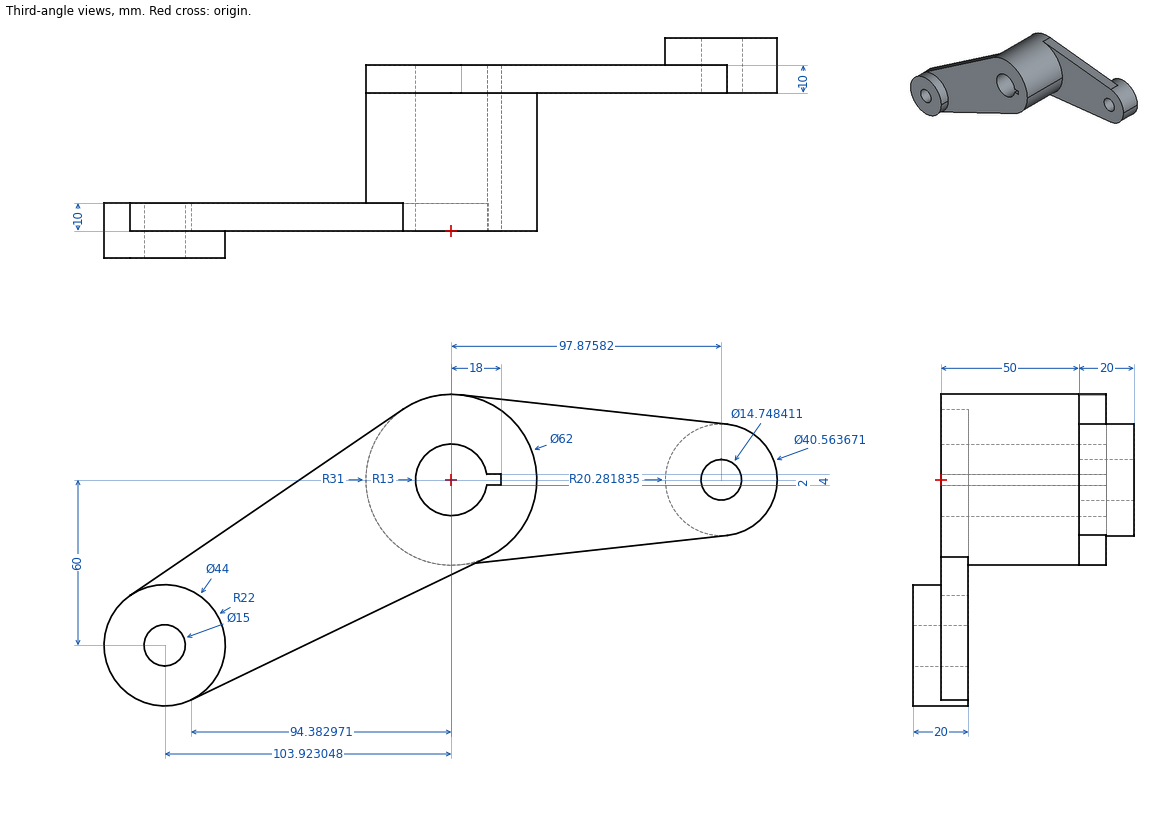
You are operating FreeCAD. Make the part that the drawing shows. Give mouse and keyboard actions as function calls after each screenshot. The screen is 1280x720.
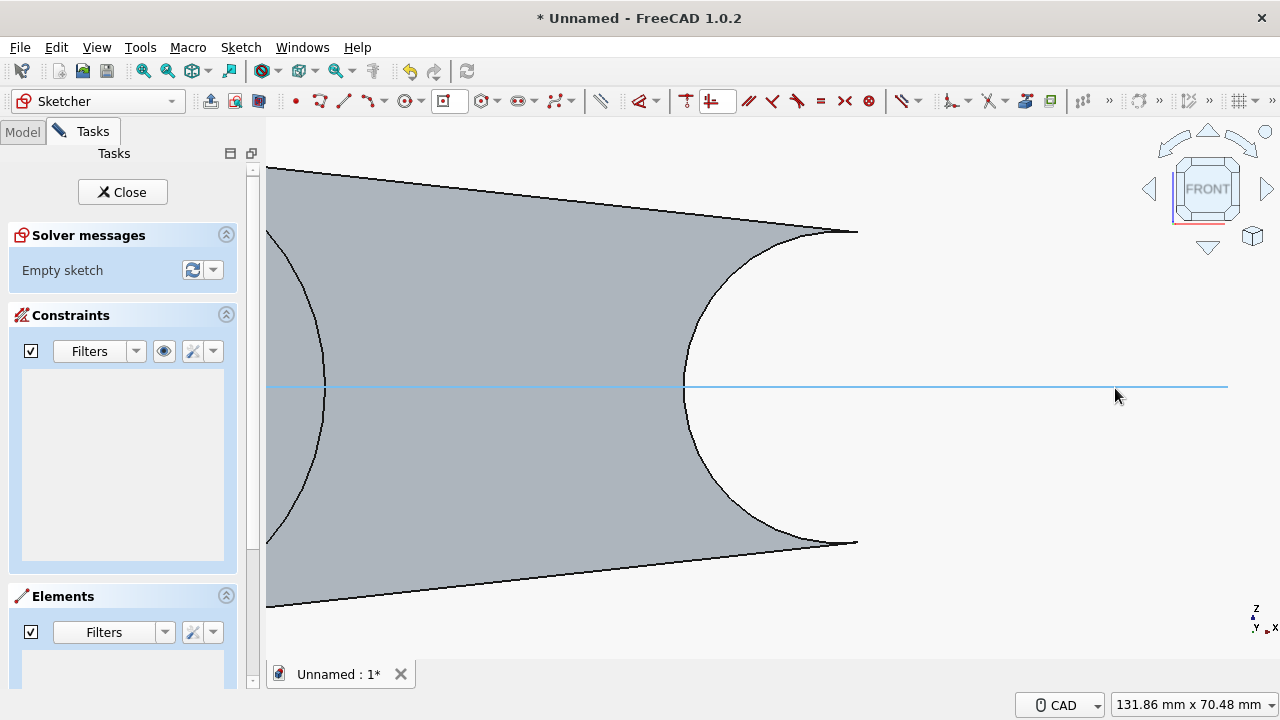
click(406, 102)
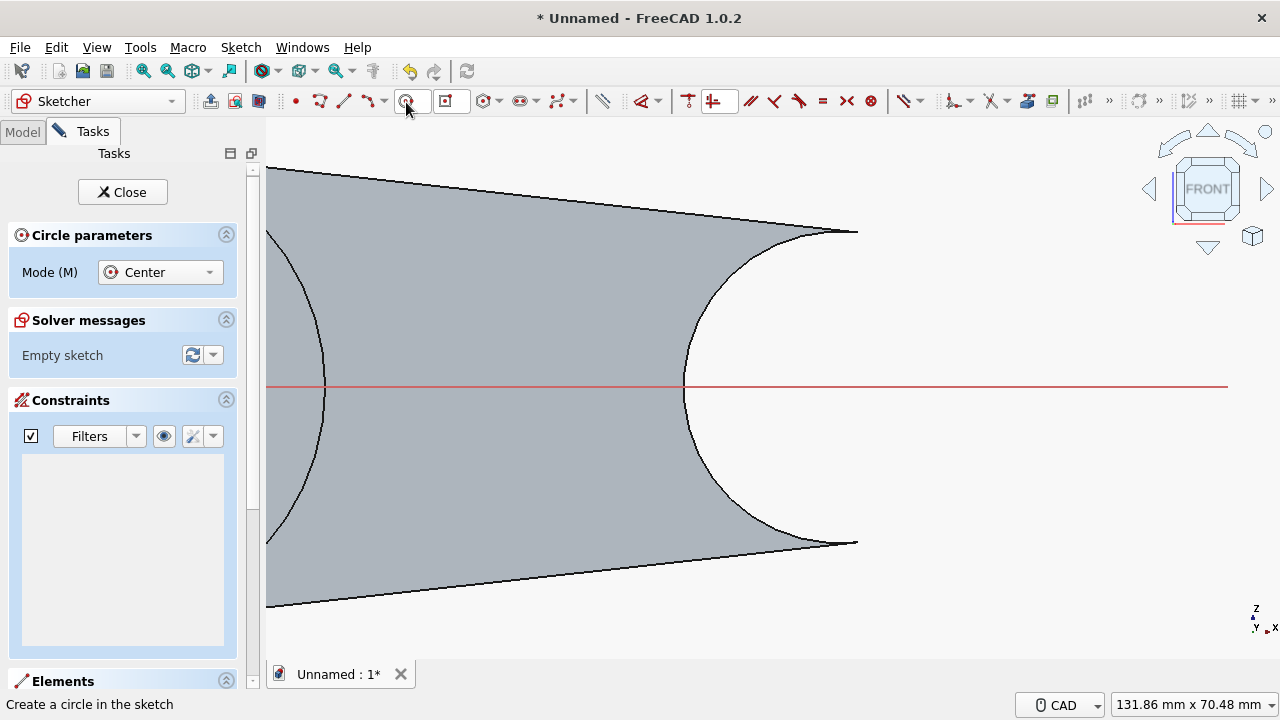
click(840, 387)
move(950, 277)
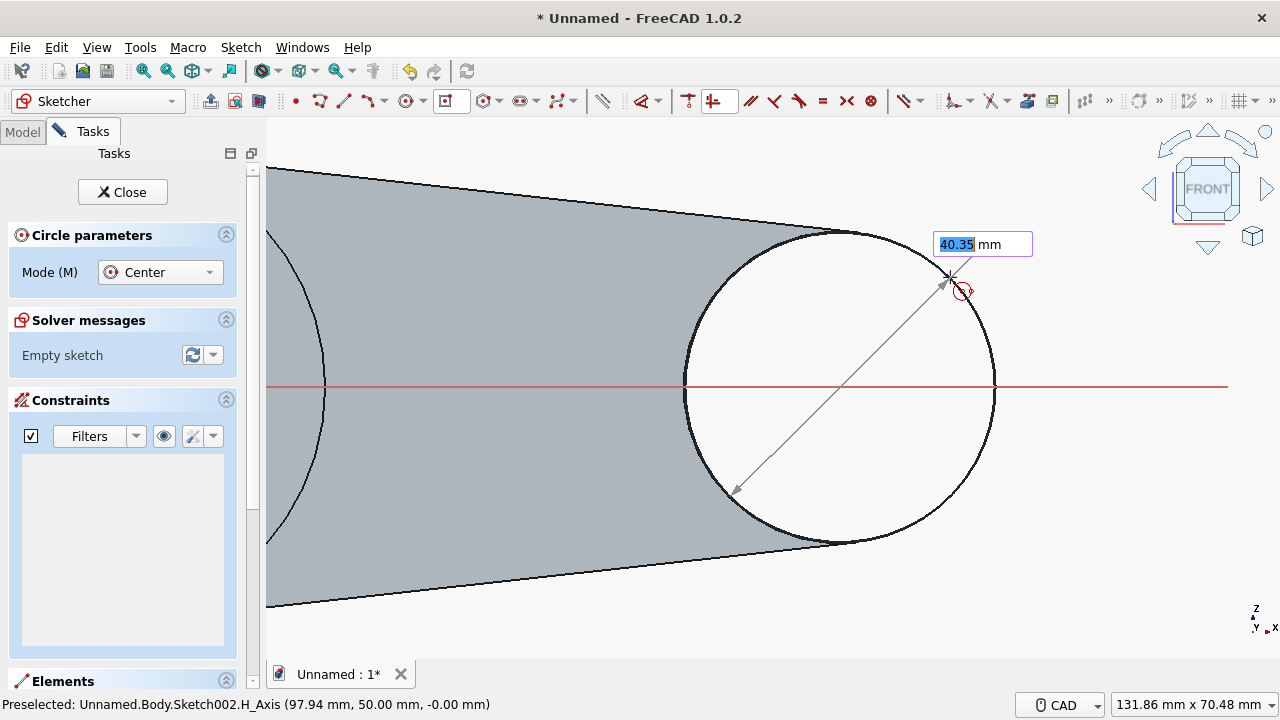
text(40.563671)
key(Return)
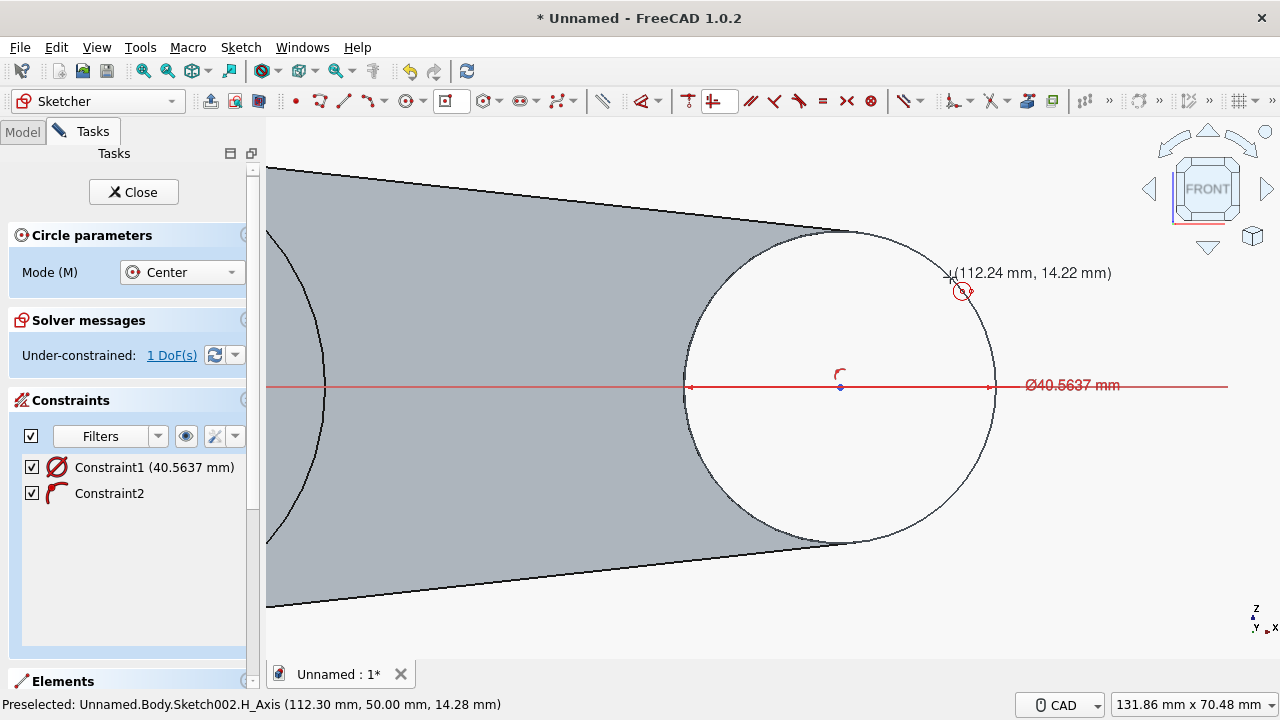
click(840, 387)
move(880, 347)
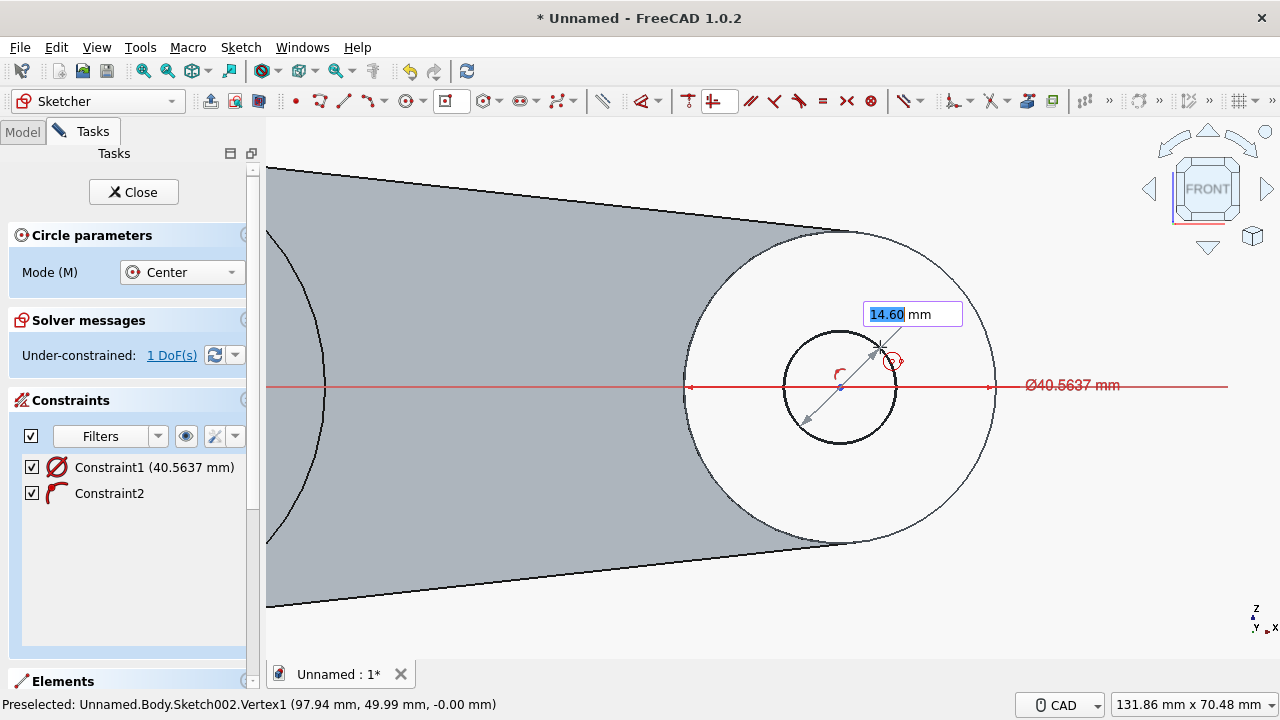
text(14.748411)
key(Return)
key(Escape)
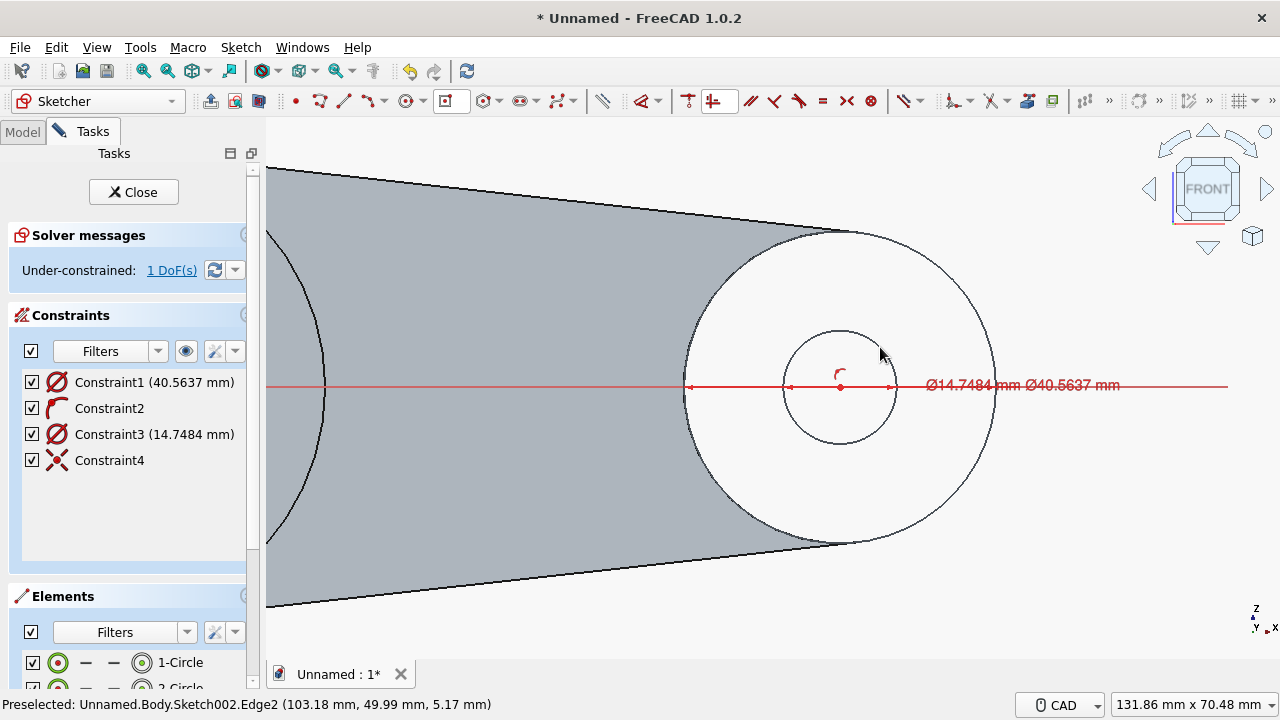
click(642, 102)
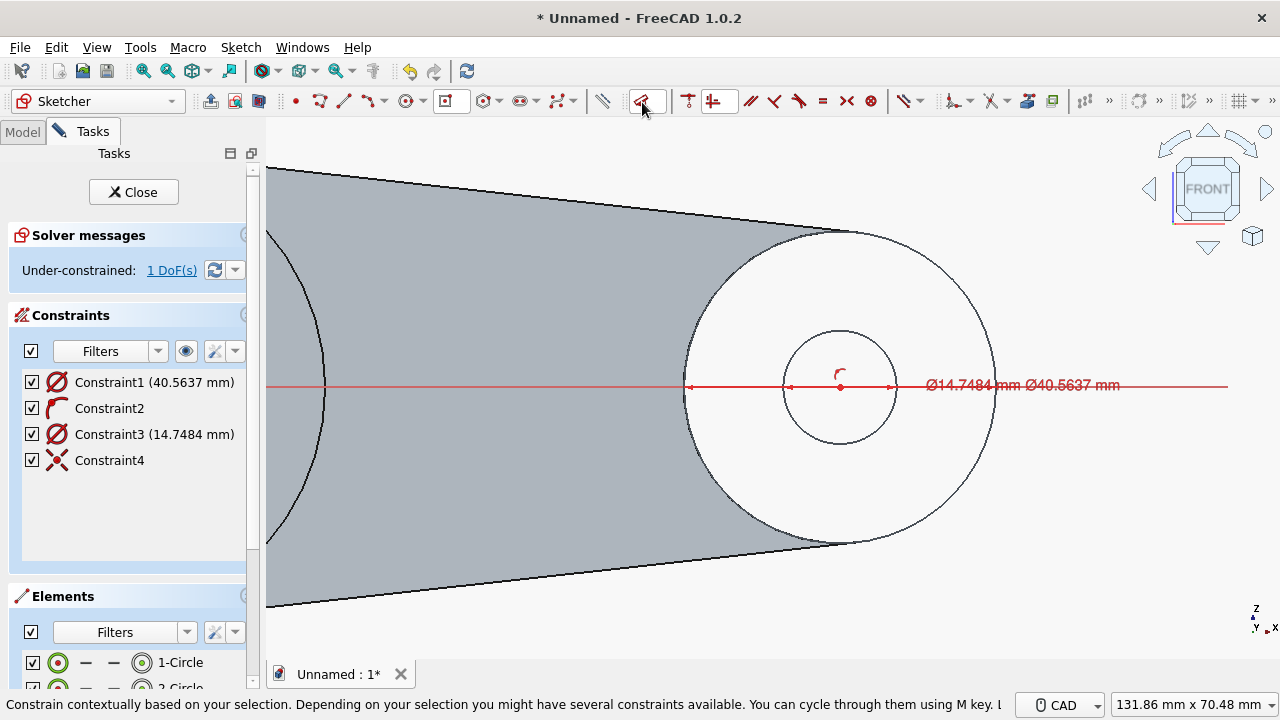
click(840, 387)
click(567, 421)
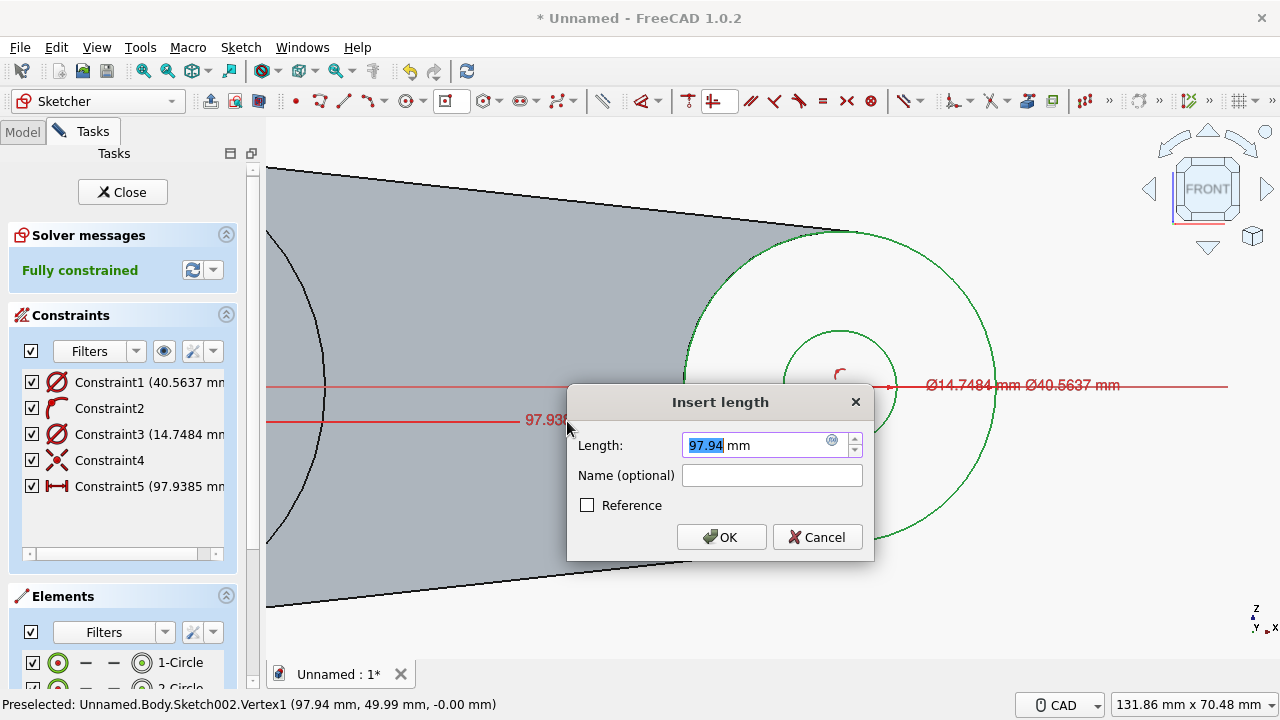
text(97.87582)
key(Return)
key(Escape)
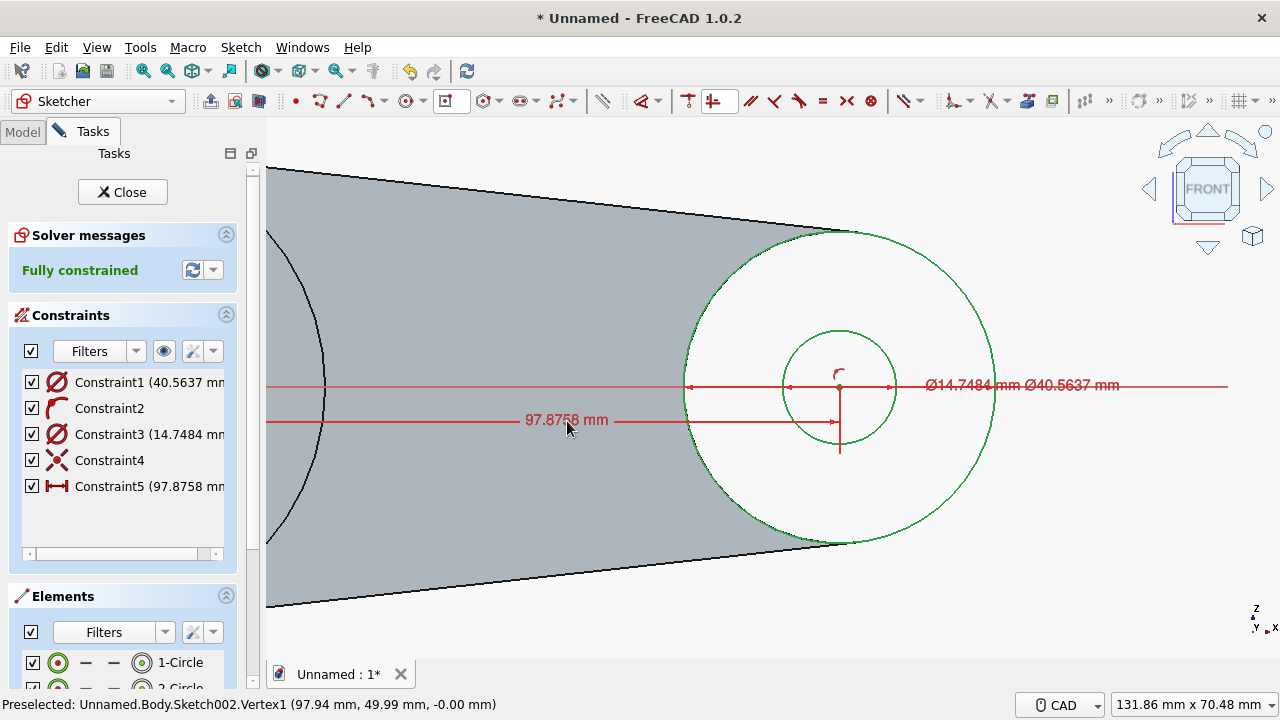
click(123, 192)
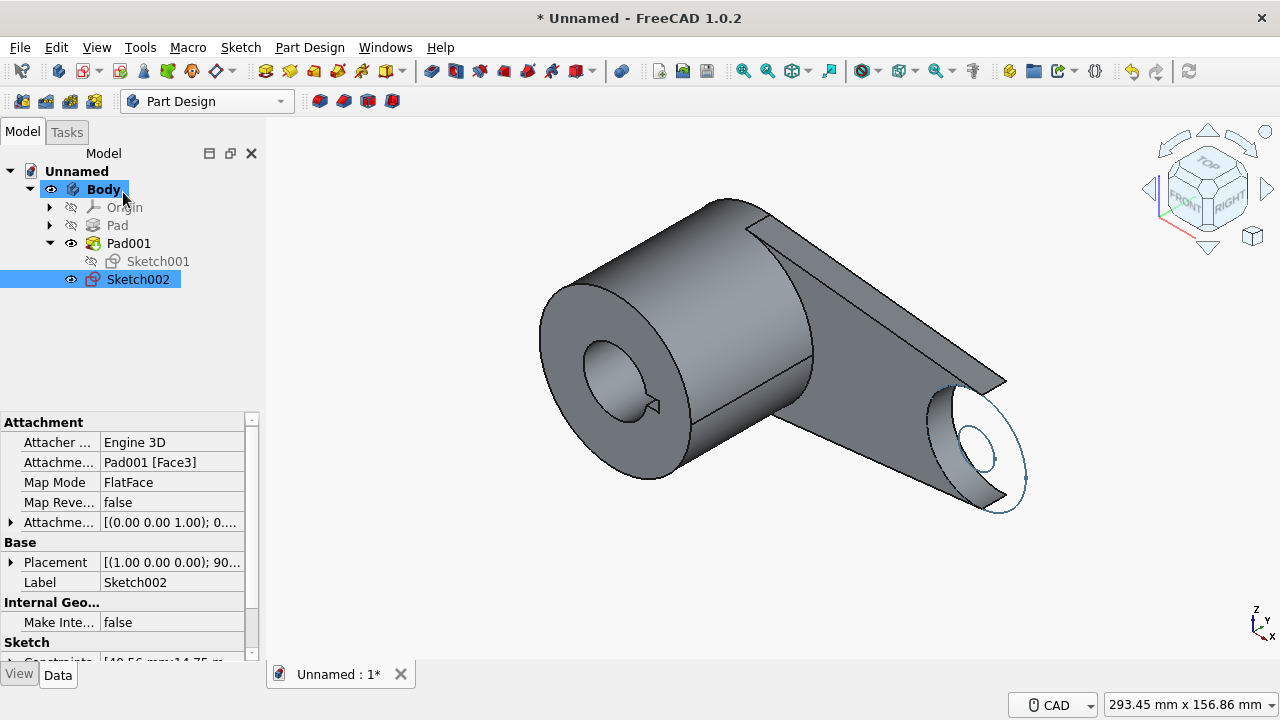
click(266, 72)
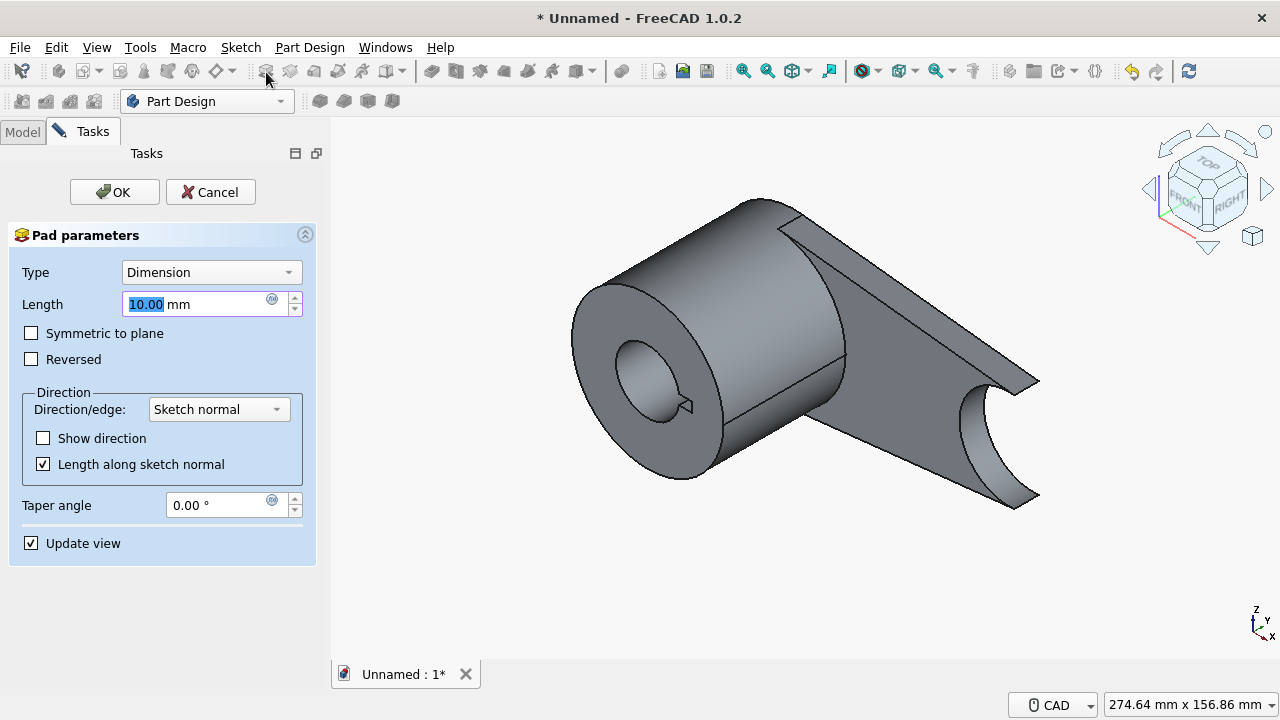
text(20)
key(Tab)